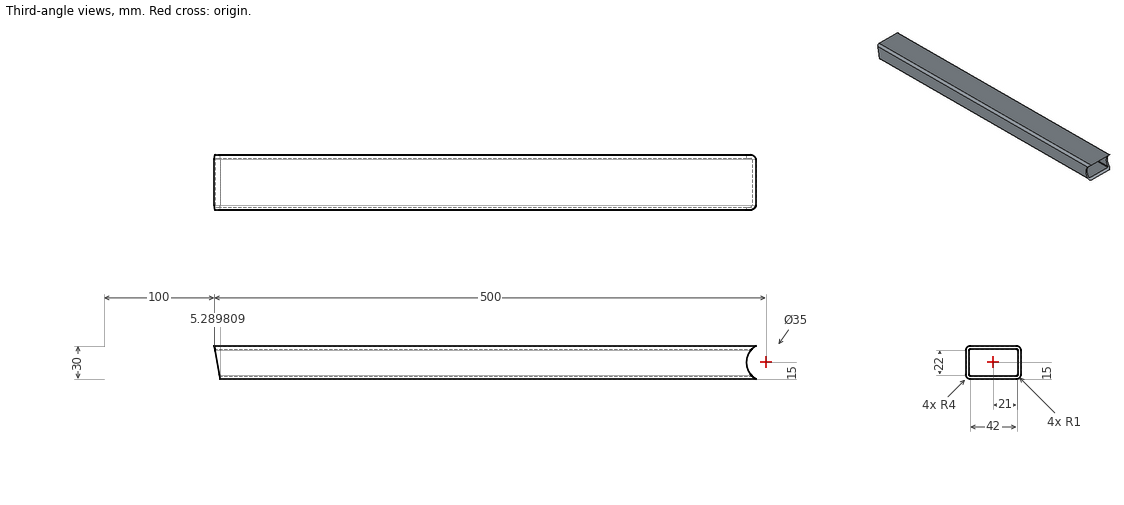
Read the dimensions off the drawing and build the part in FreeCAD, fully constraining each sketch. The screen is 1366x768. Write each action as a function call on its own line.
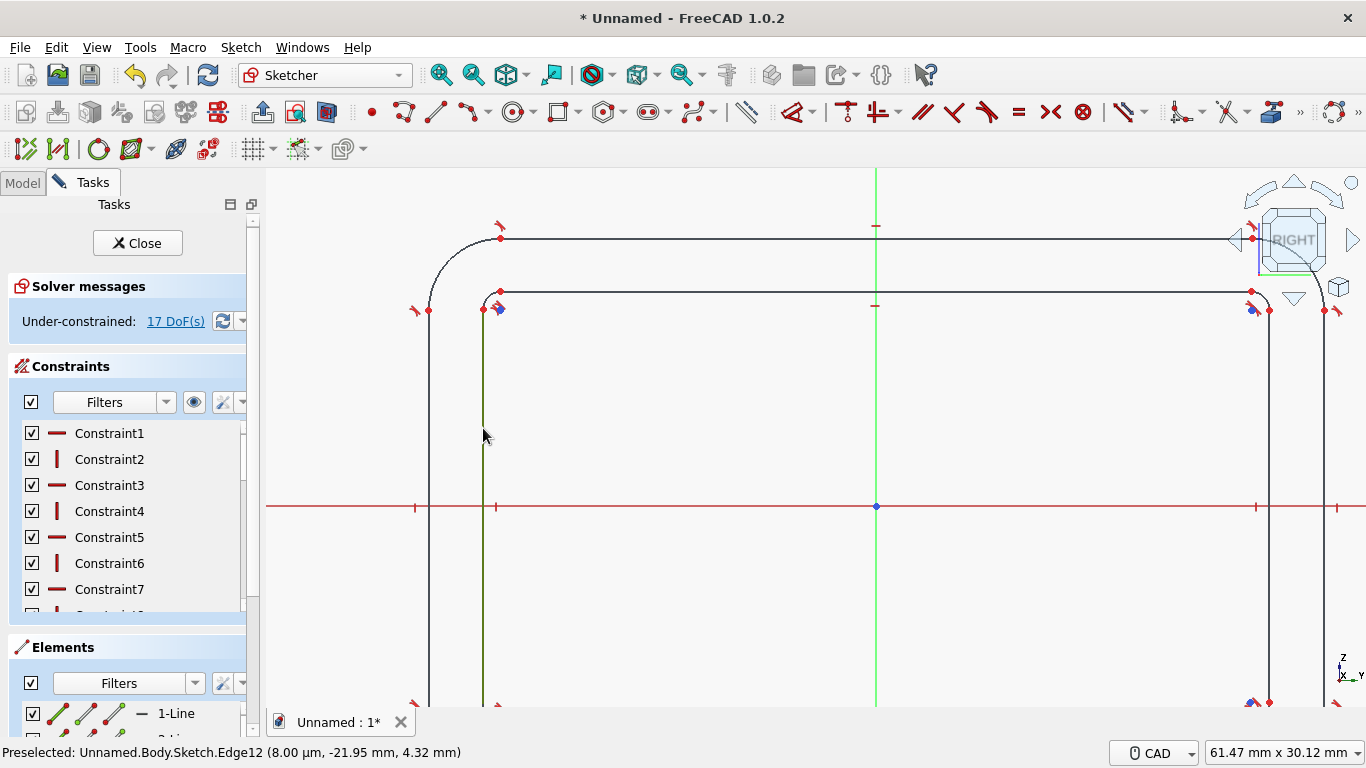
scroll(486, 298, down, 2)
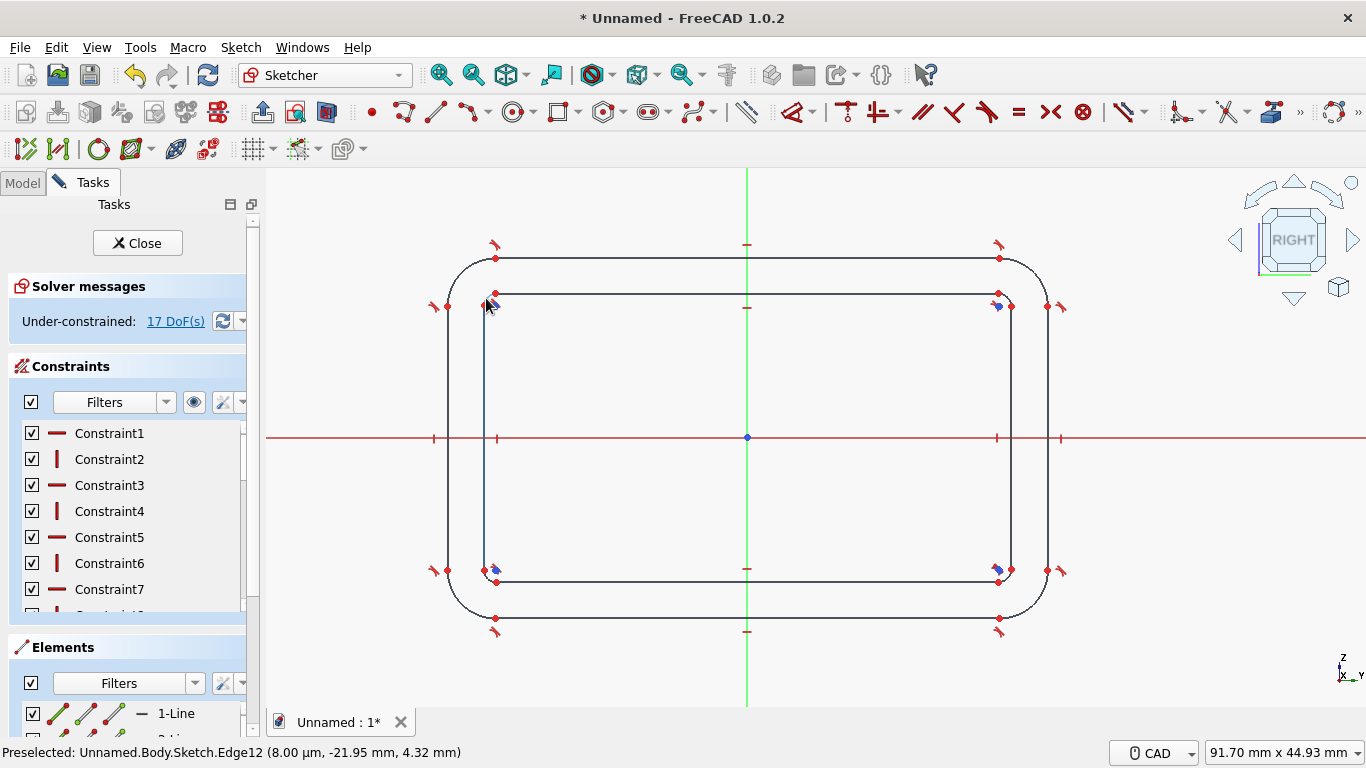
scroll(488, 579, up, 3)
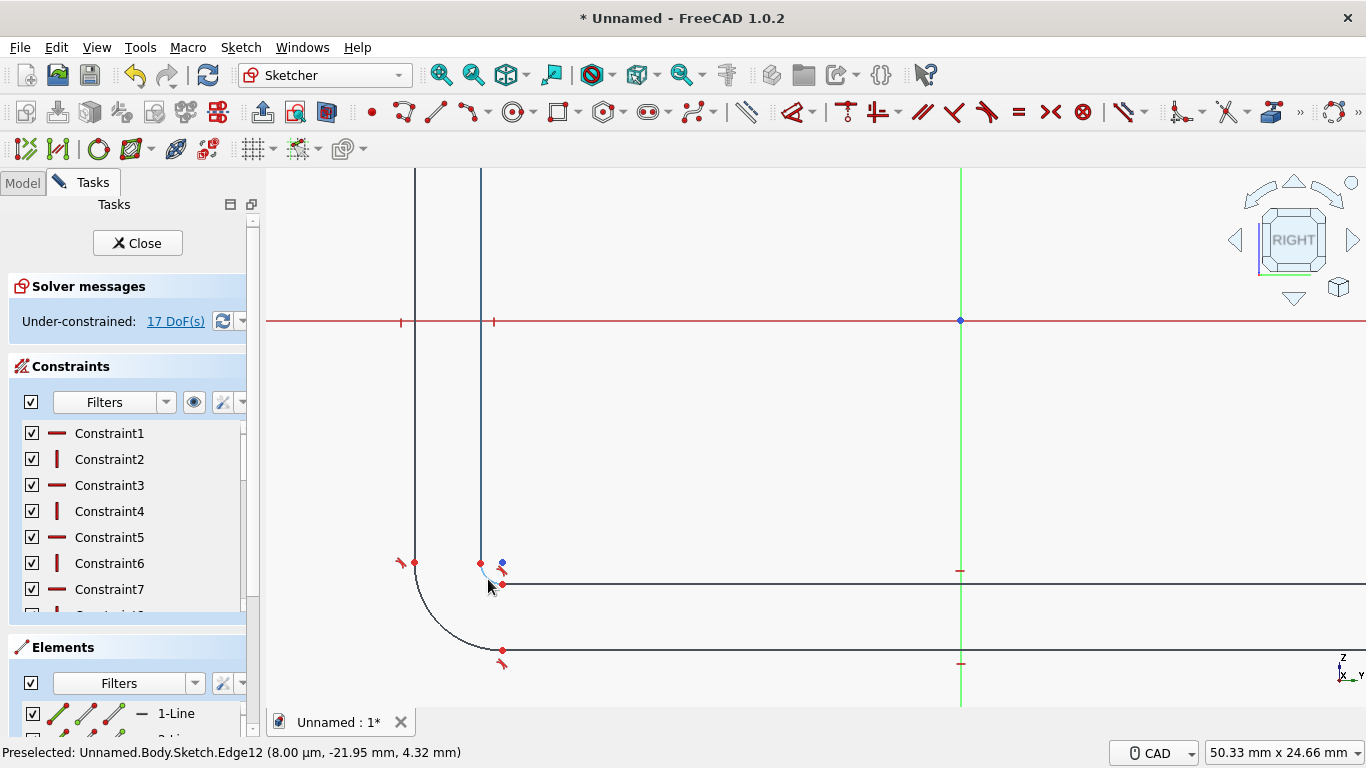
click(487, 578)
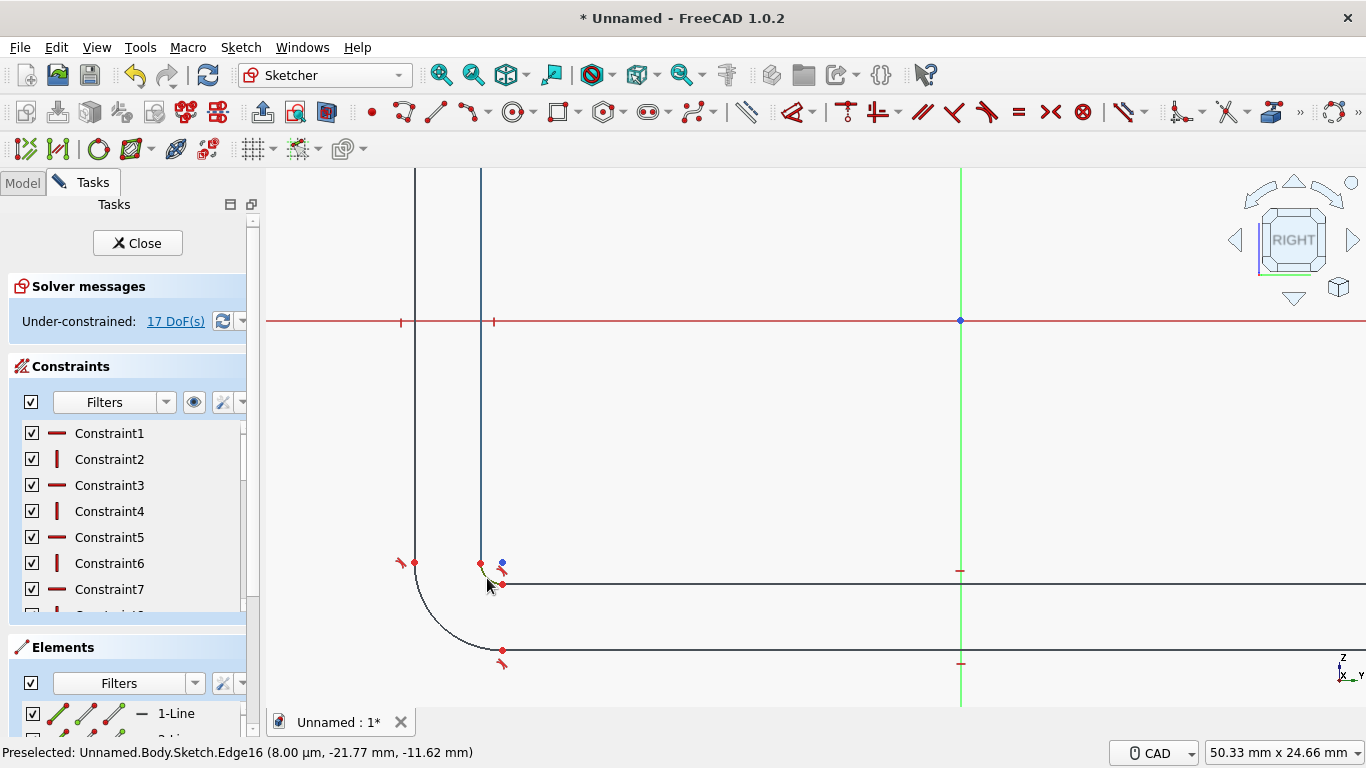
click(988, 112)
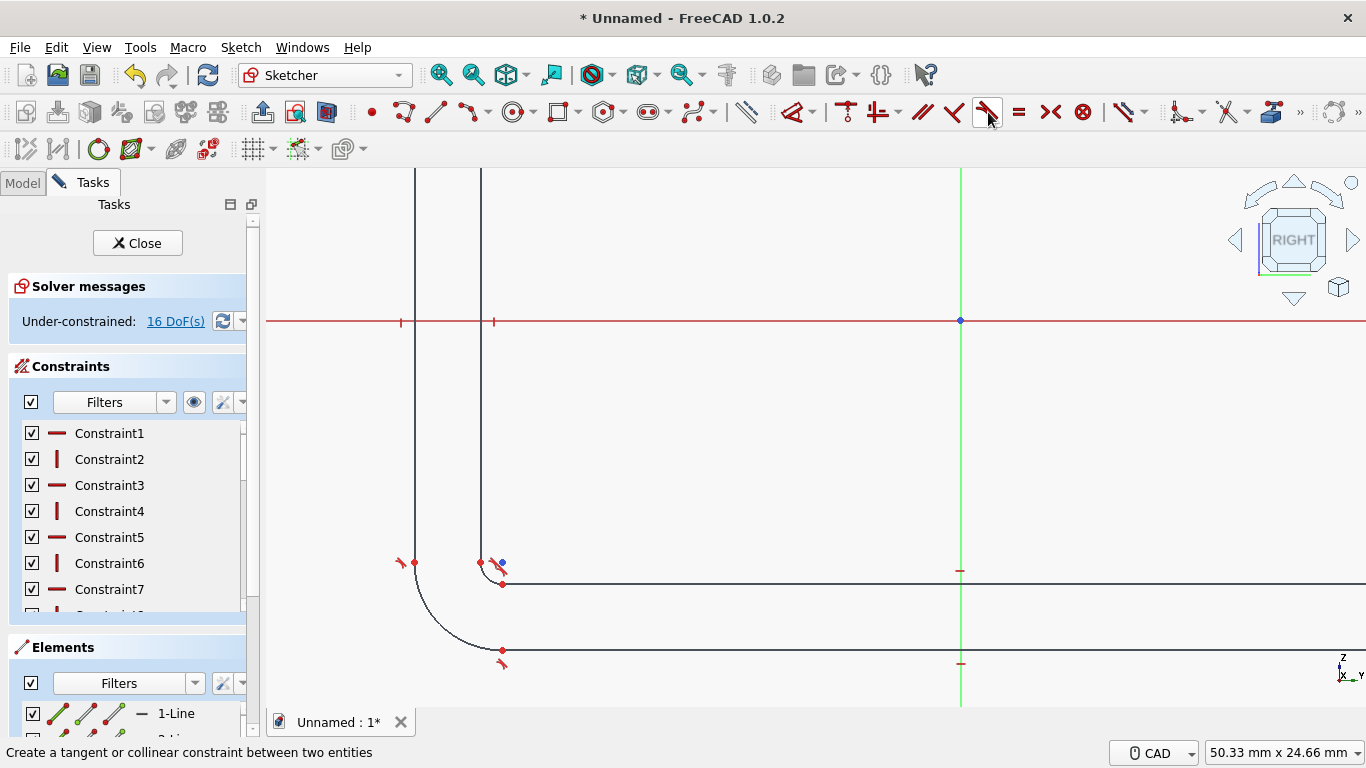
scroll(488, 579, down, 3)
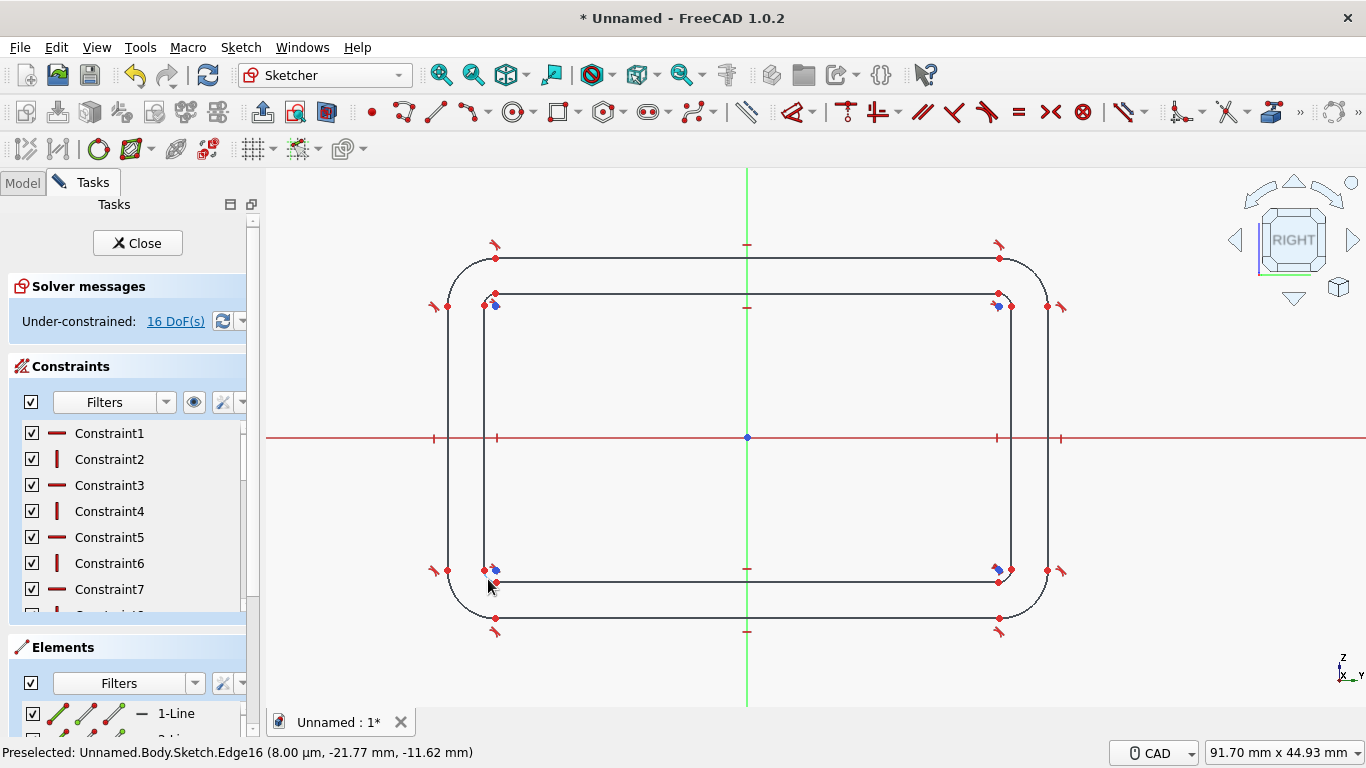
click(1022, 613)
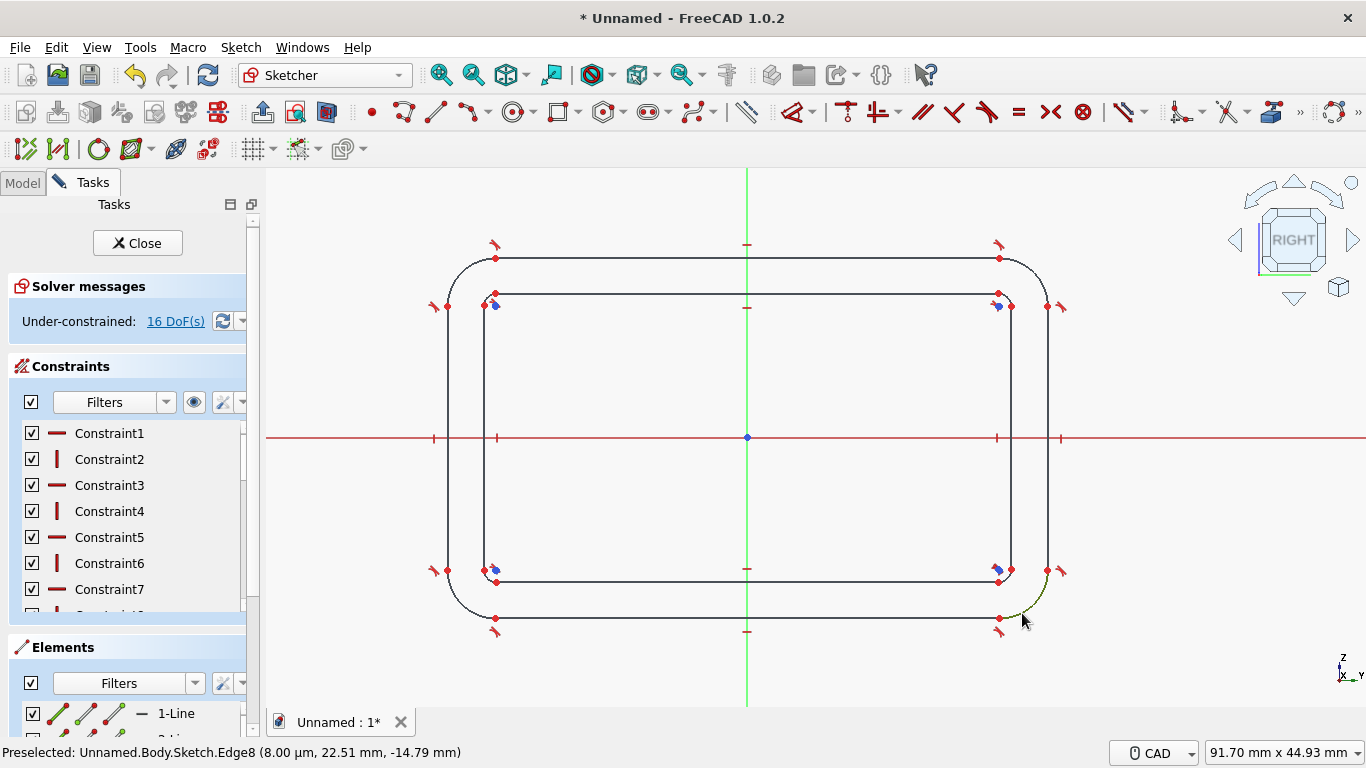
scroll(1007, 578, up, 2)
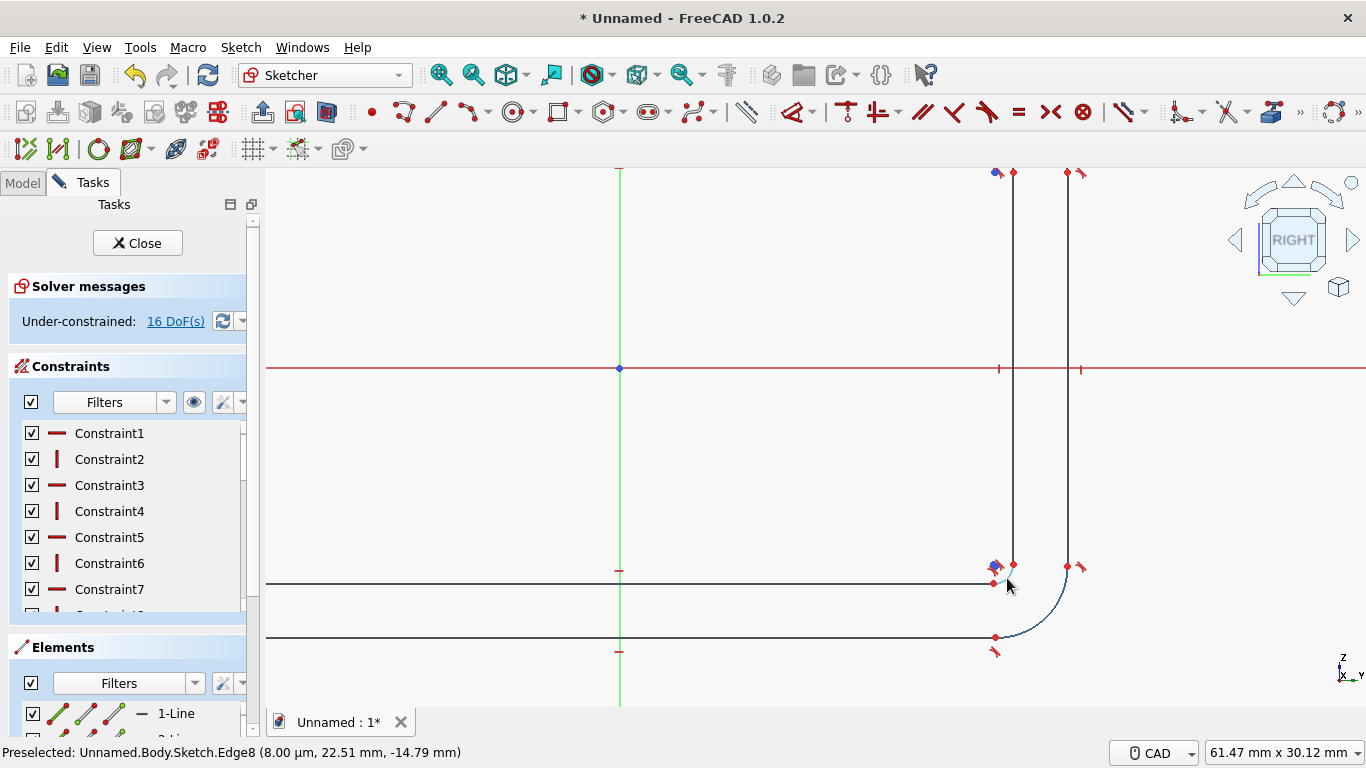
click(1007, 578)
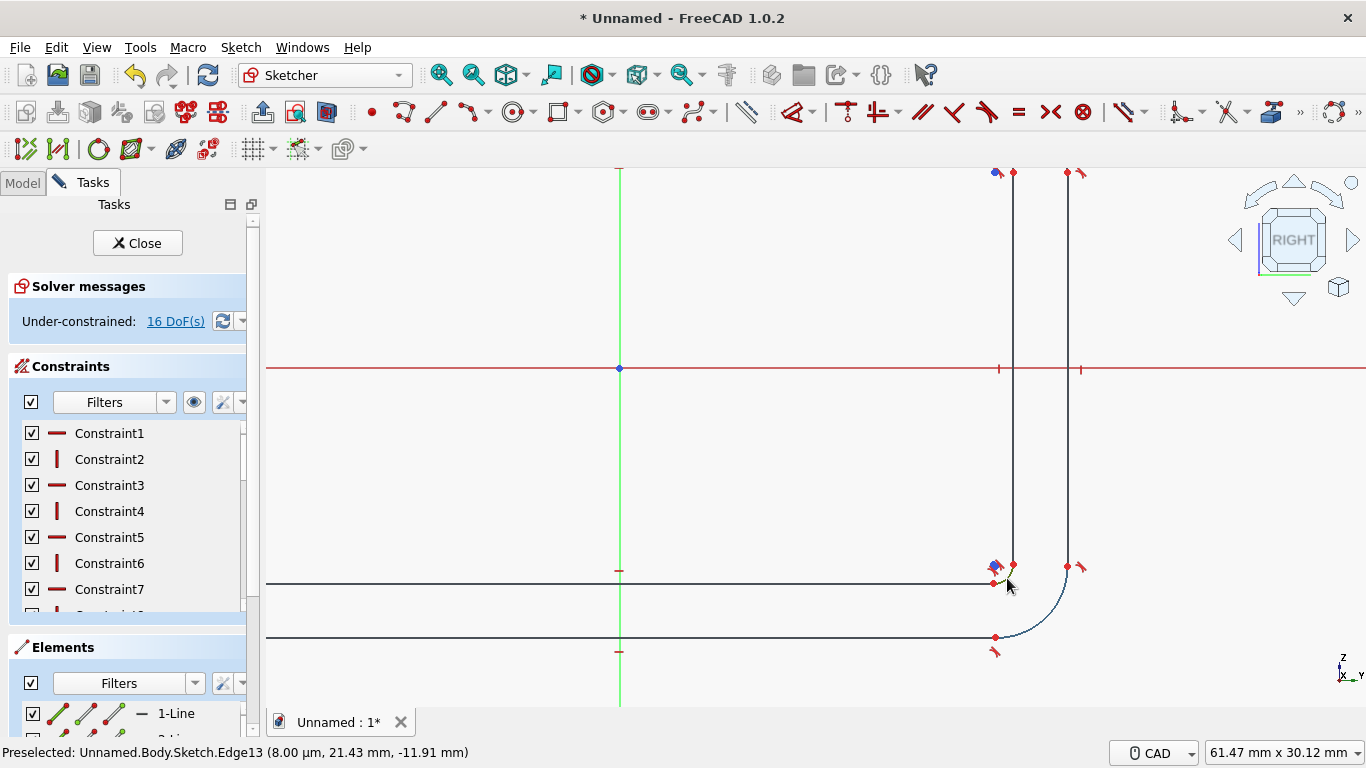
key(c)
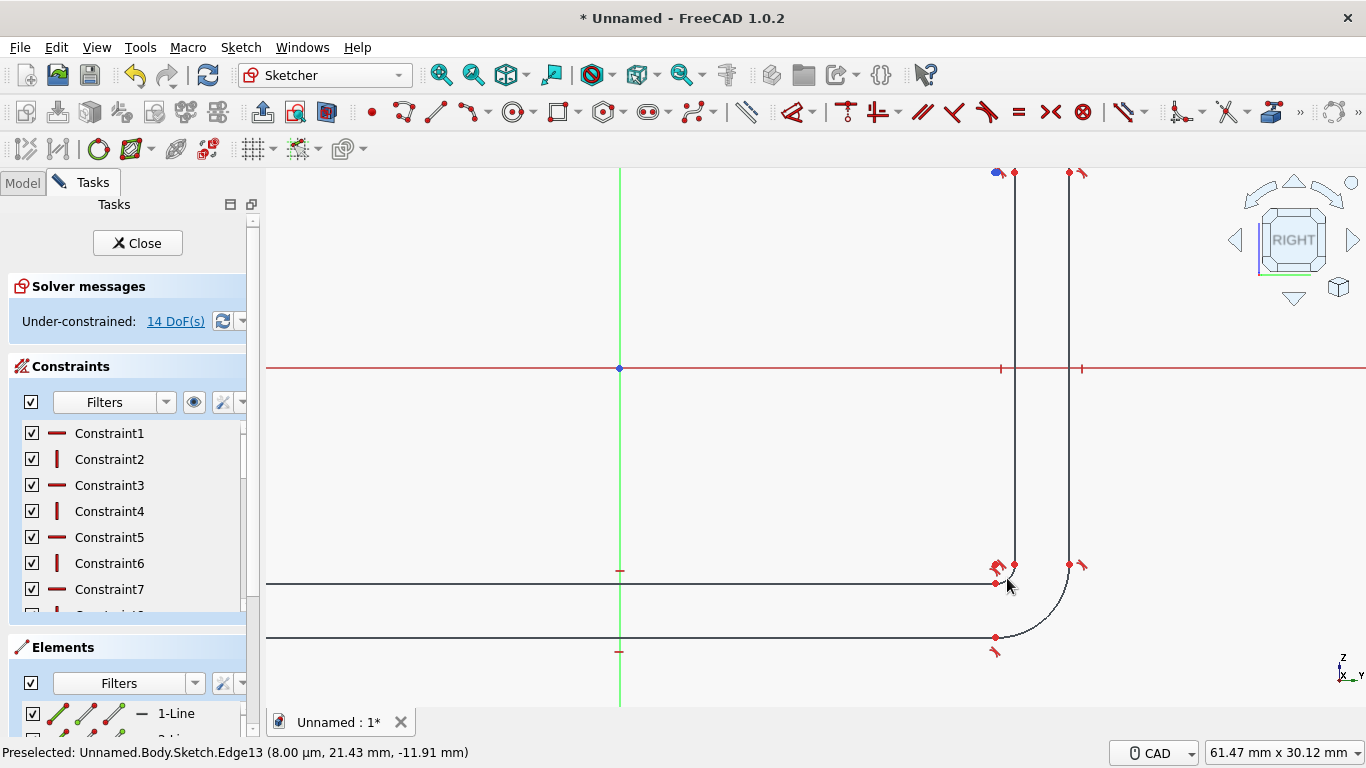
scroll(1008, 578, down, 2)